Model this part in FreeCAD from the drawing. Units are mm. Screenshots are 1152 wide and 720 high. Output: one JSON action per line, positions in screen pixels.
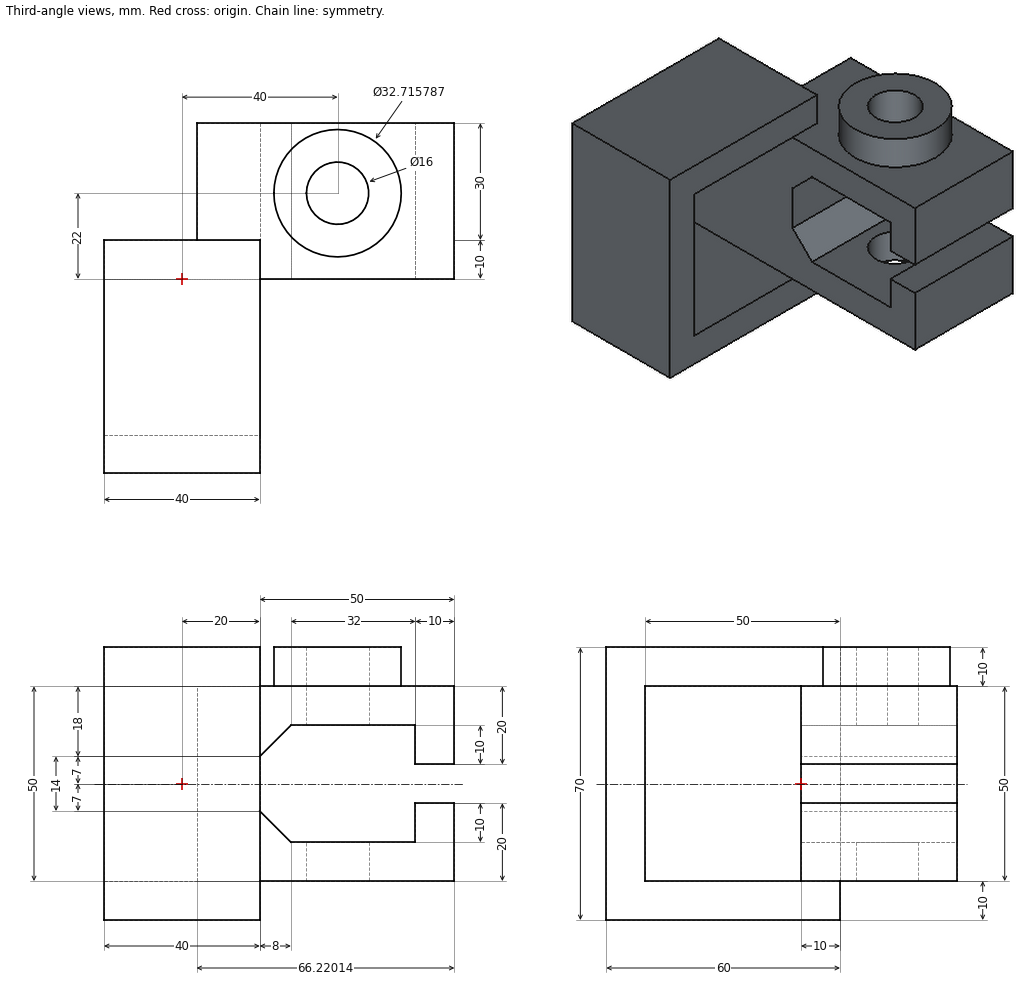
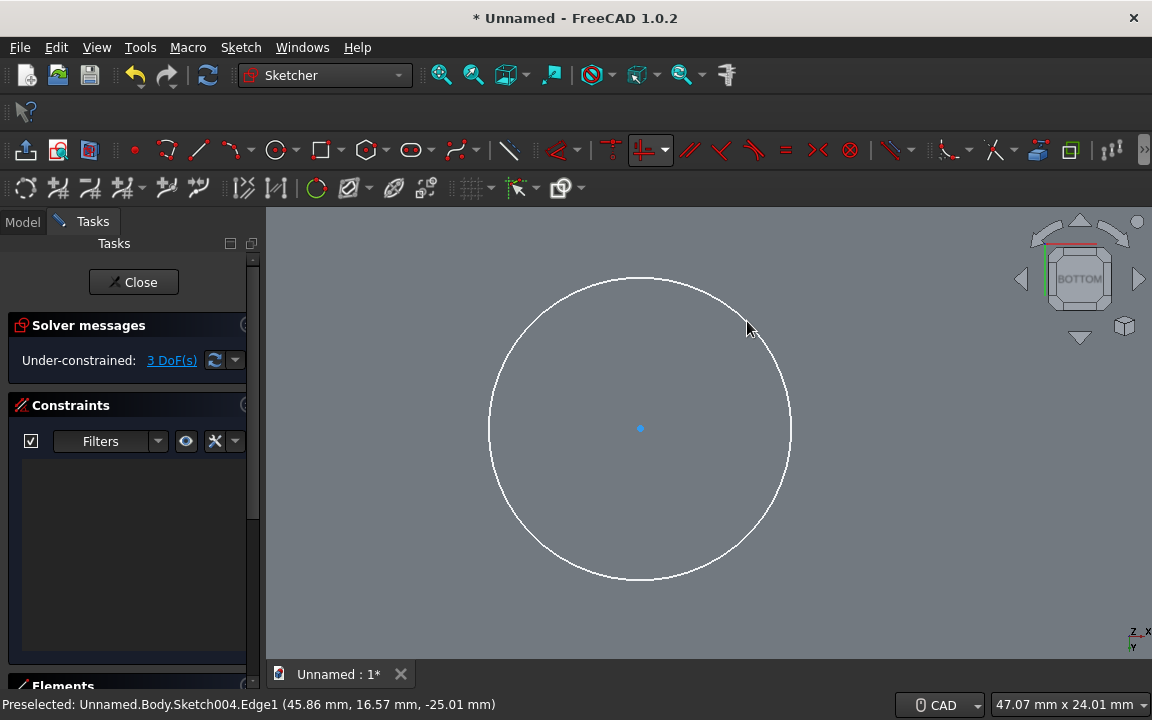
{"action": "key", "text": "d"}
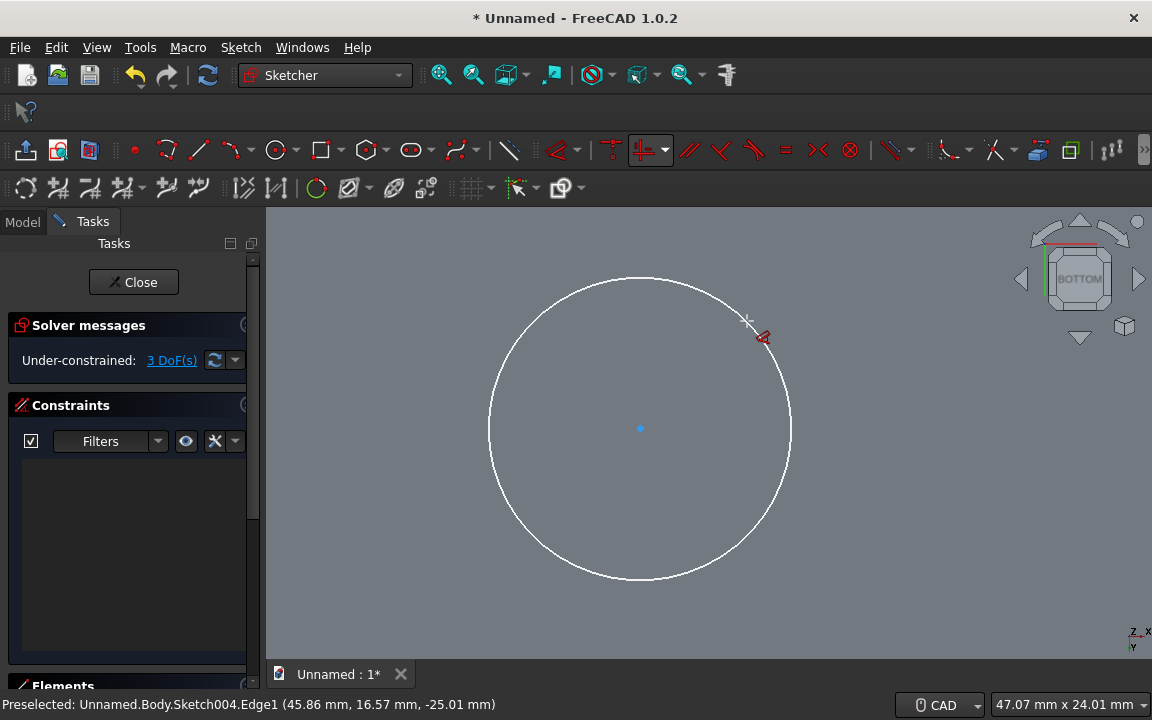
{"action": "left_click", "coordinate": [747, 322]}
{"action": "left_click", "coordinate": [770, 299]}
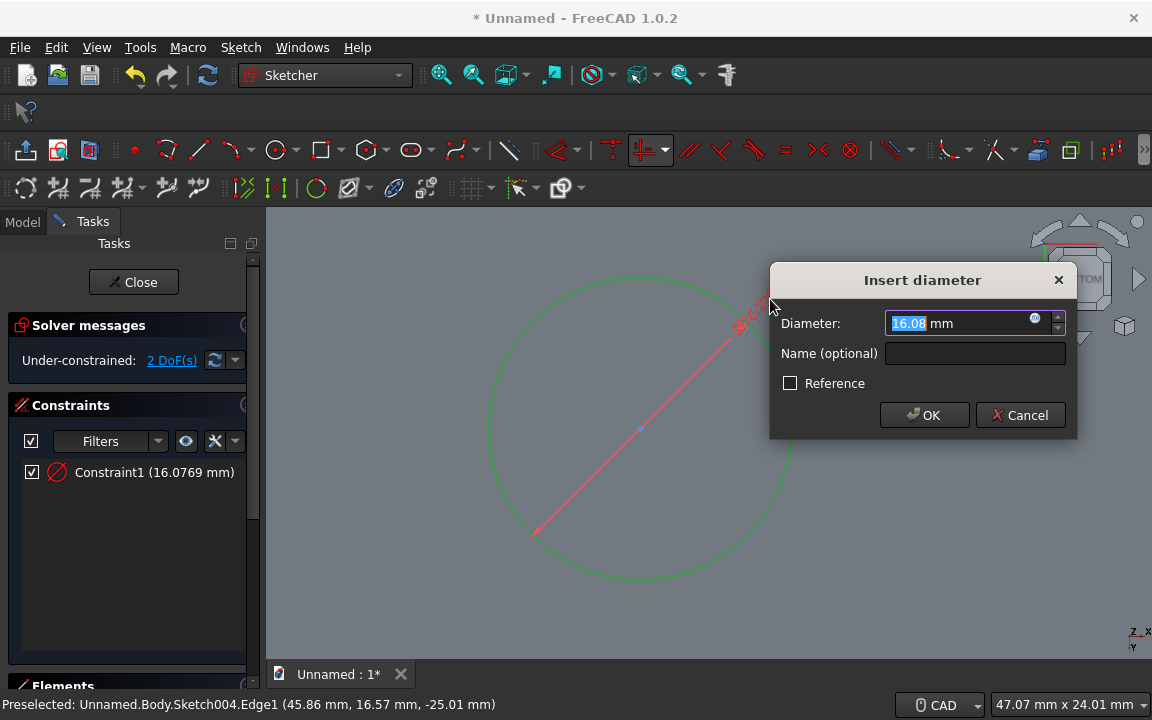
{"action": "type", "text": "16"}
{"action": "key", "text": "Return"}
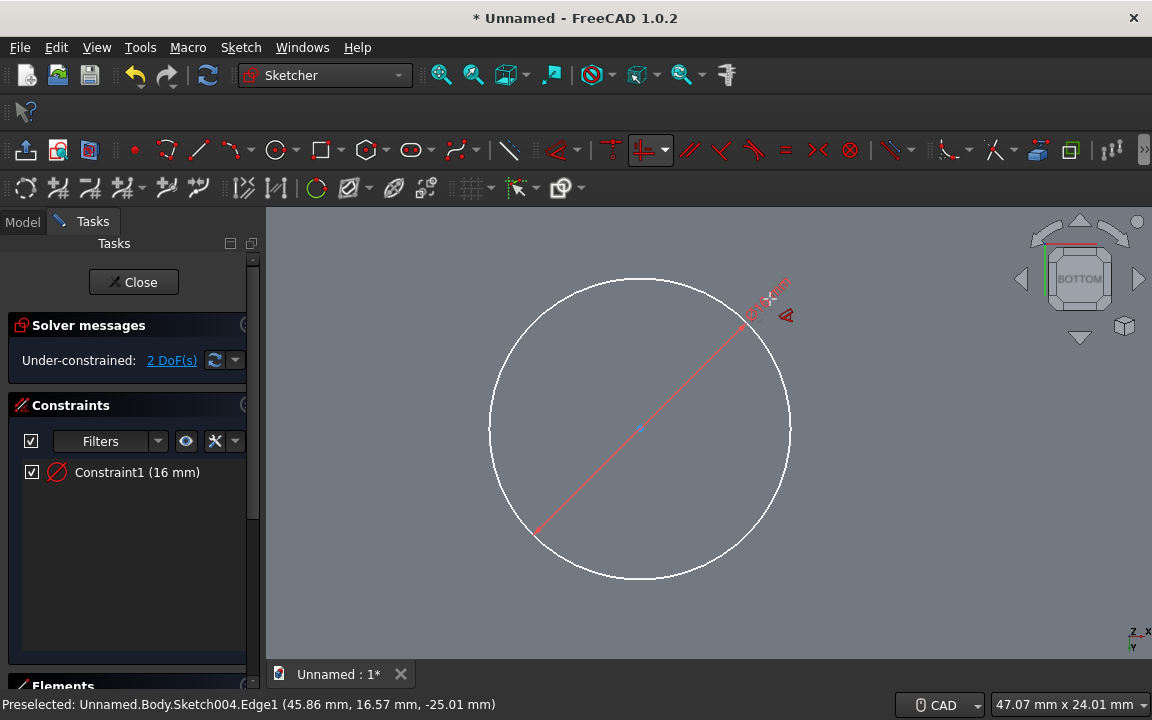
{"action": "left_click", "coordinate": [640, 429]}
{"action": "left_click", "coordinate": [467, 463]}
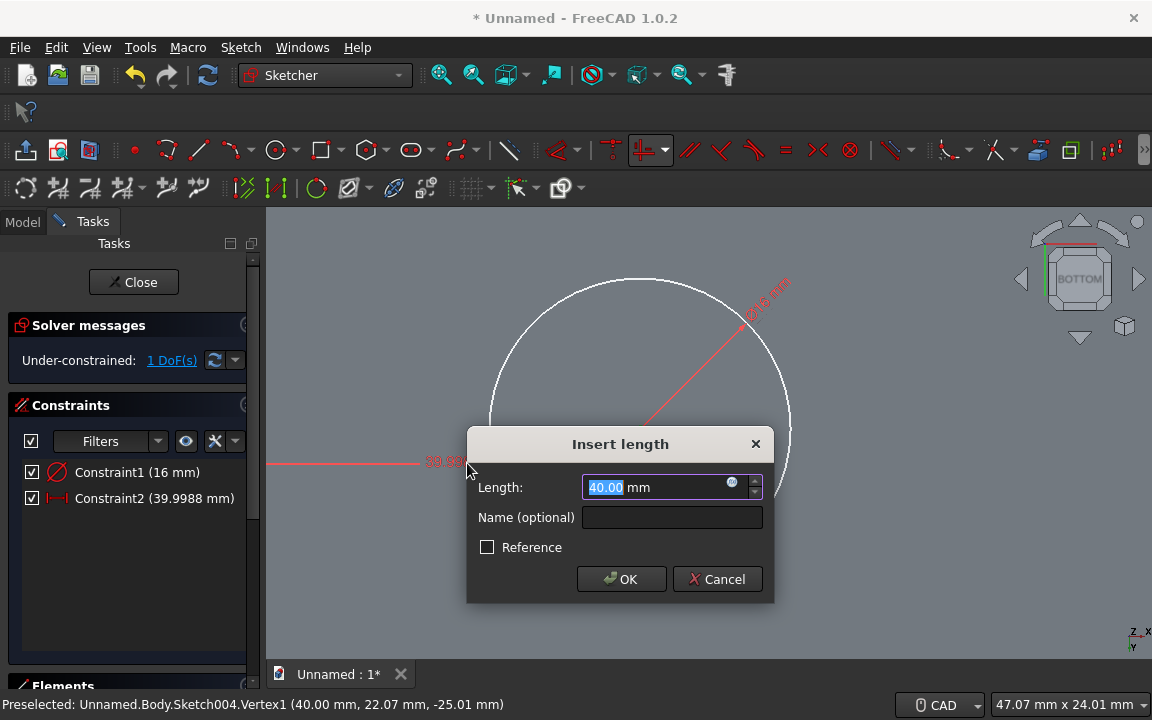
{"action": "type", "text": "40"}
{"action": "key", "text": "Return"}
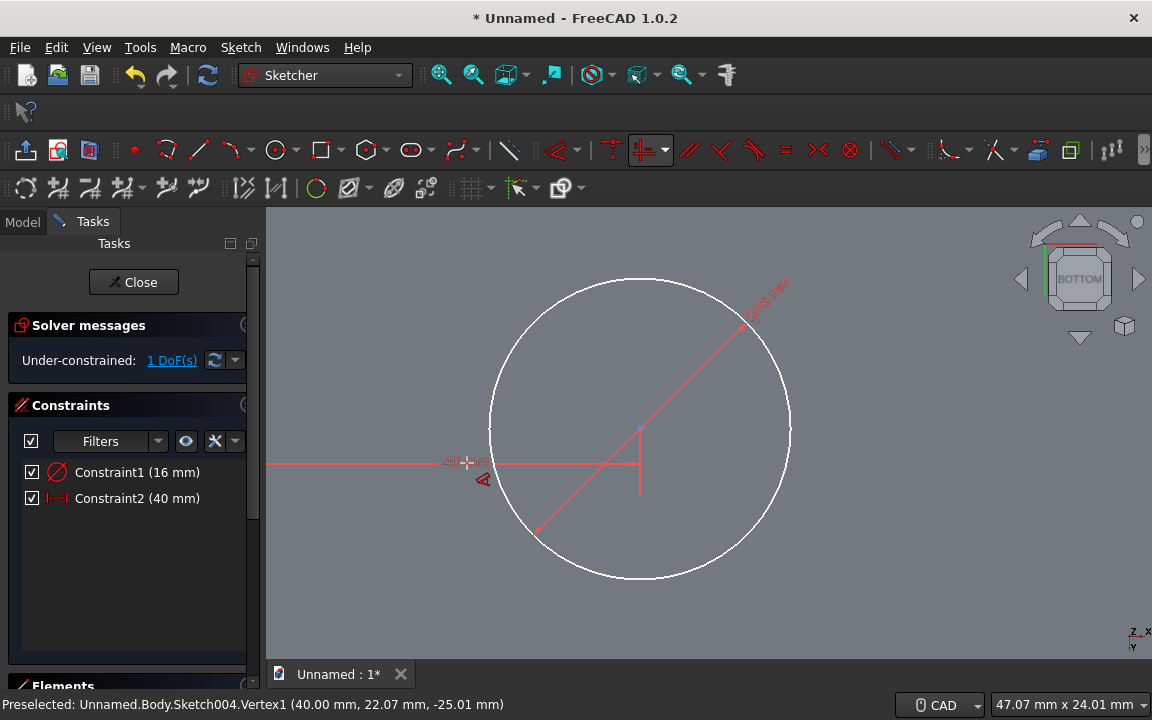
{"action": "left_click", "coordinate": [640, 429]}
{"action": "left_click", "coordinate": [674, 332]}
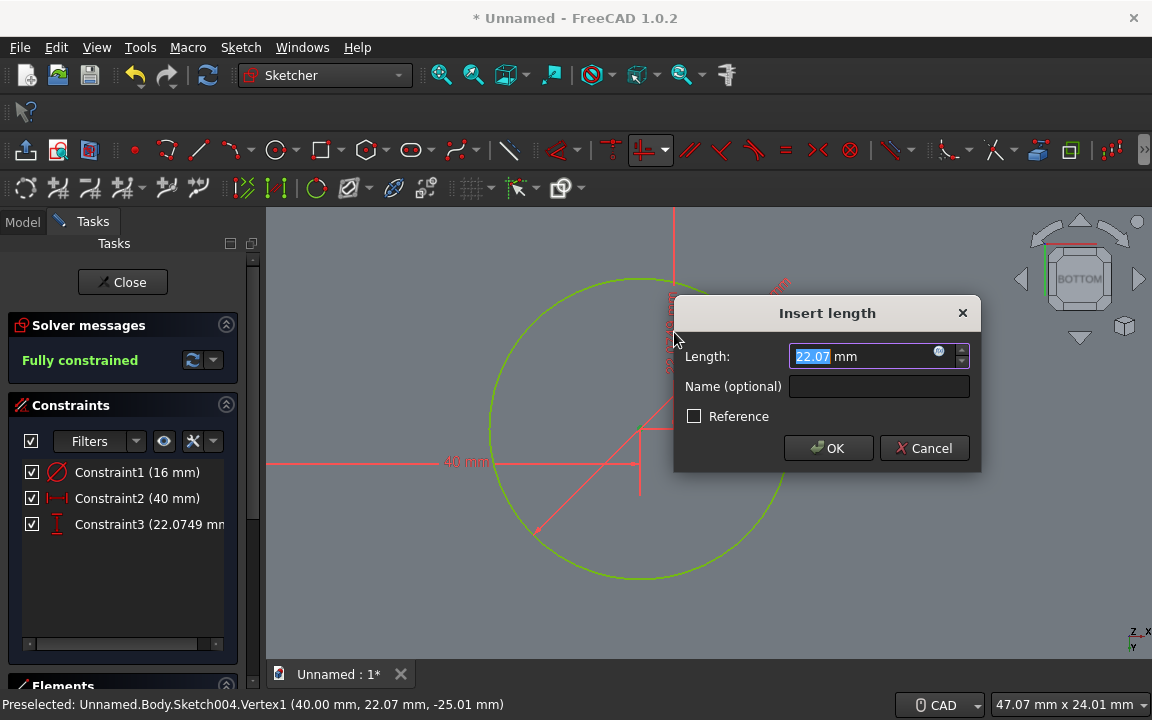
{"action": "type", "text": "22"}
{"action": "key", "text": "Return"}
{"action": "key", "text": "Escape"}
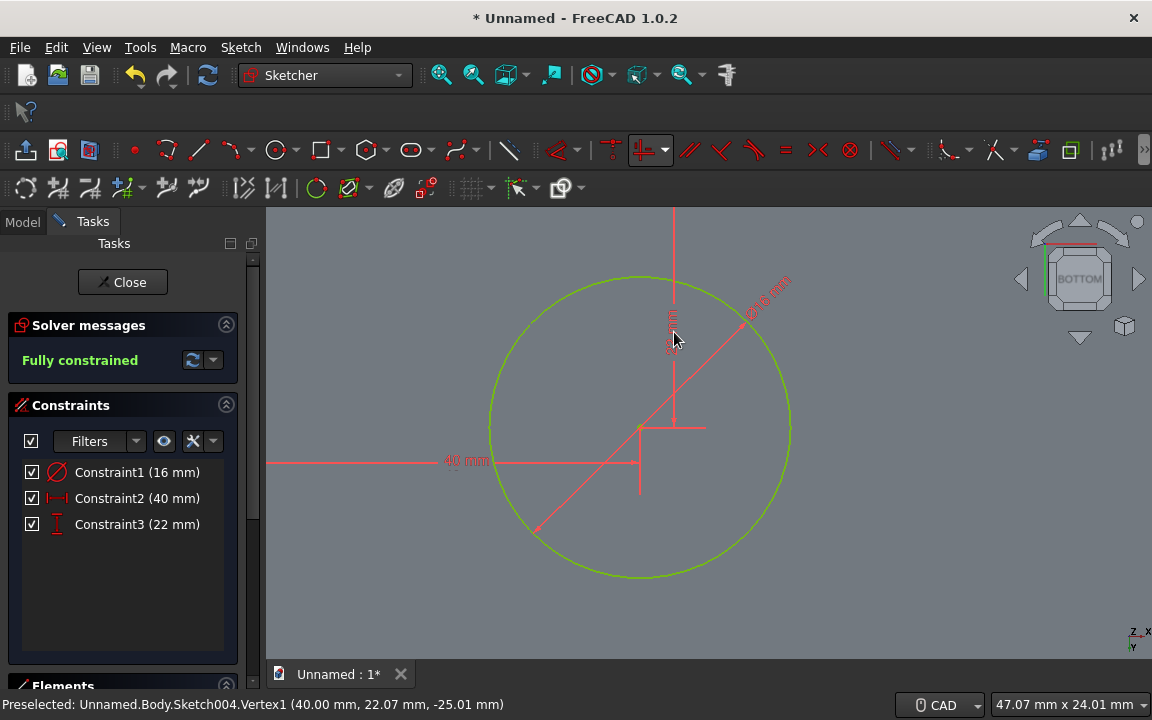
{"action": "left_click", "coordinate": [123, 282]}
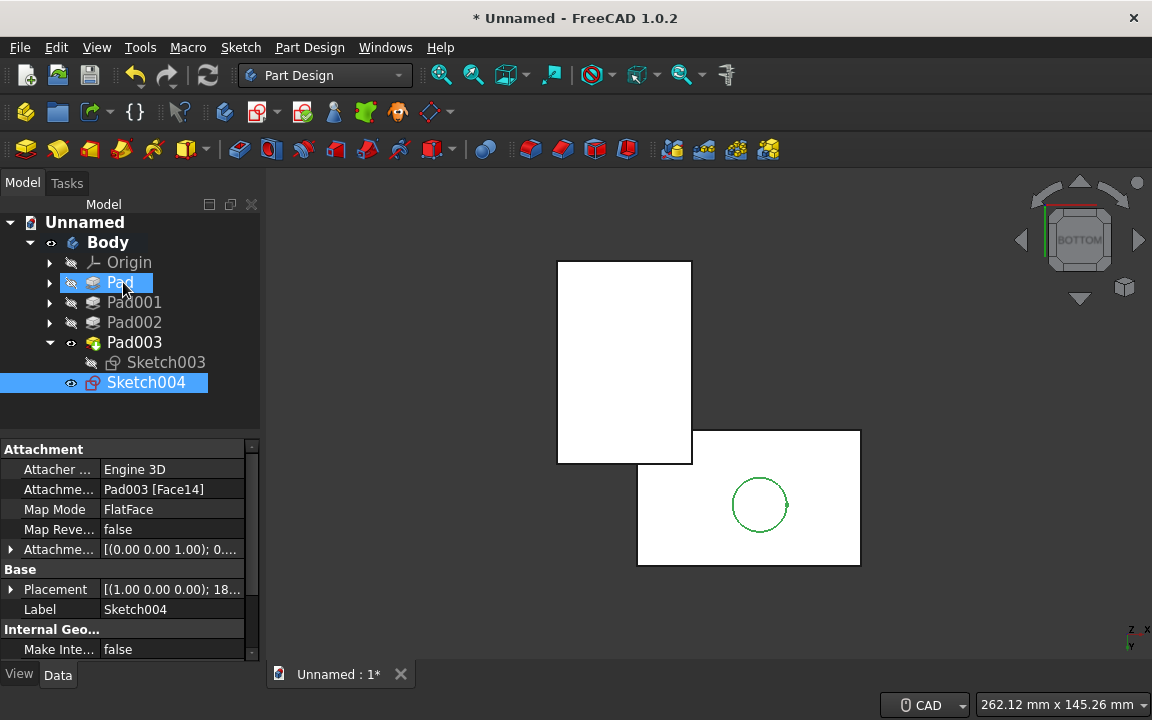
{"action": "left_click", "coordinate": [240, 150]}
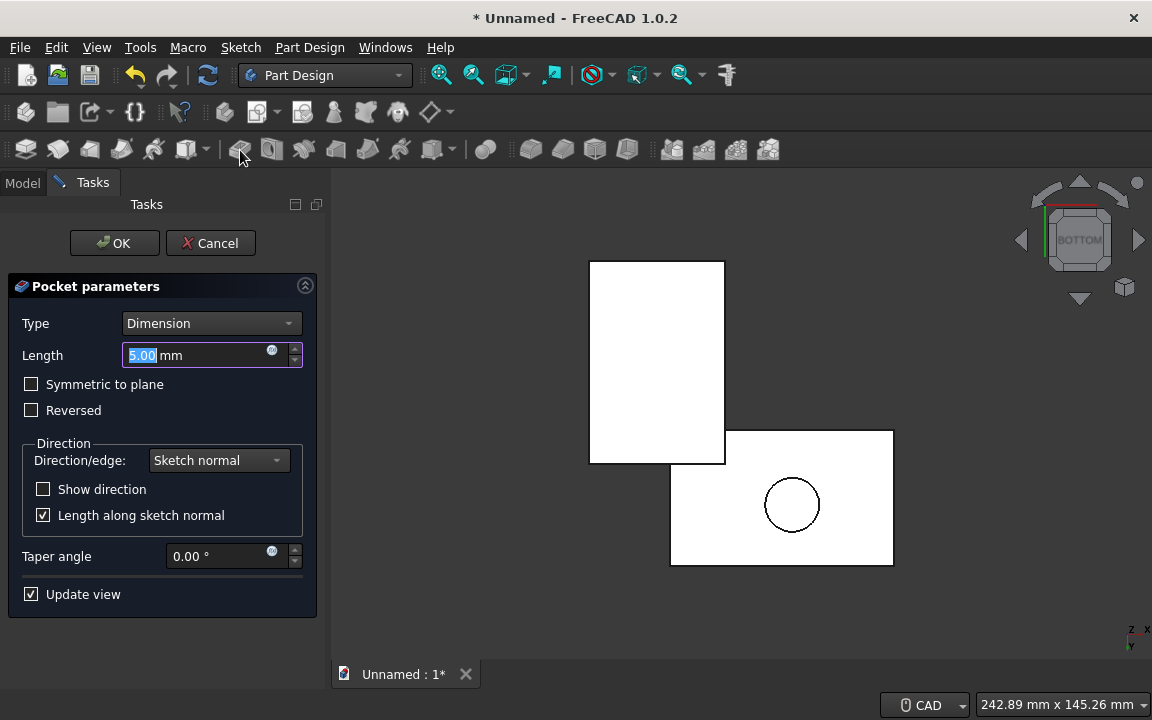
{"action": "type", "text": "50"}
{"action": "key", "text": "Tab"}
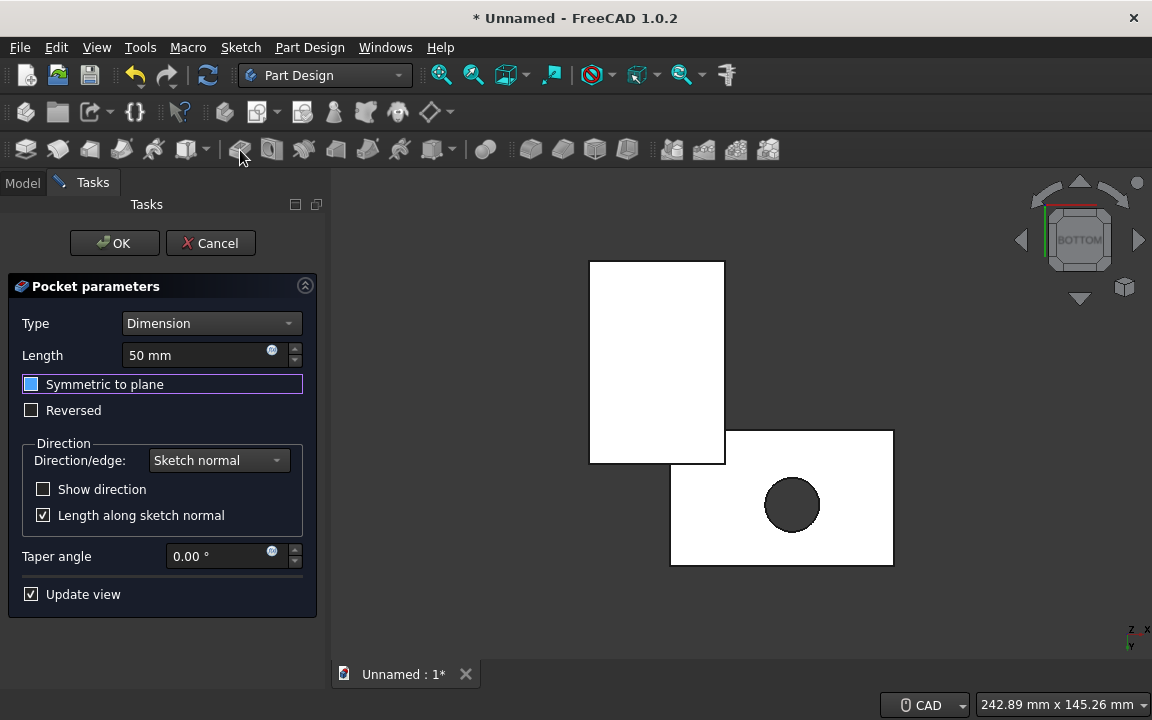
{"action": "left_click", "coordinate": [115, 243]}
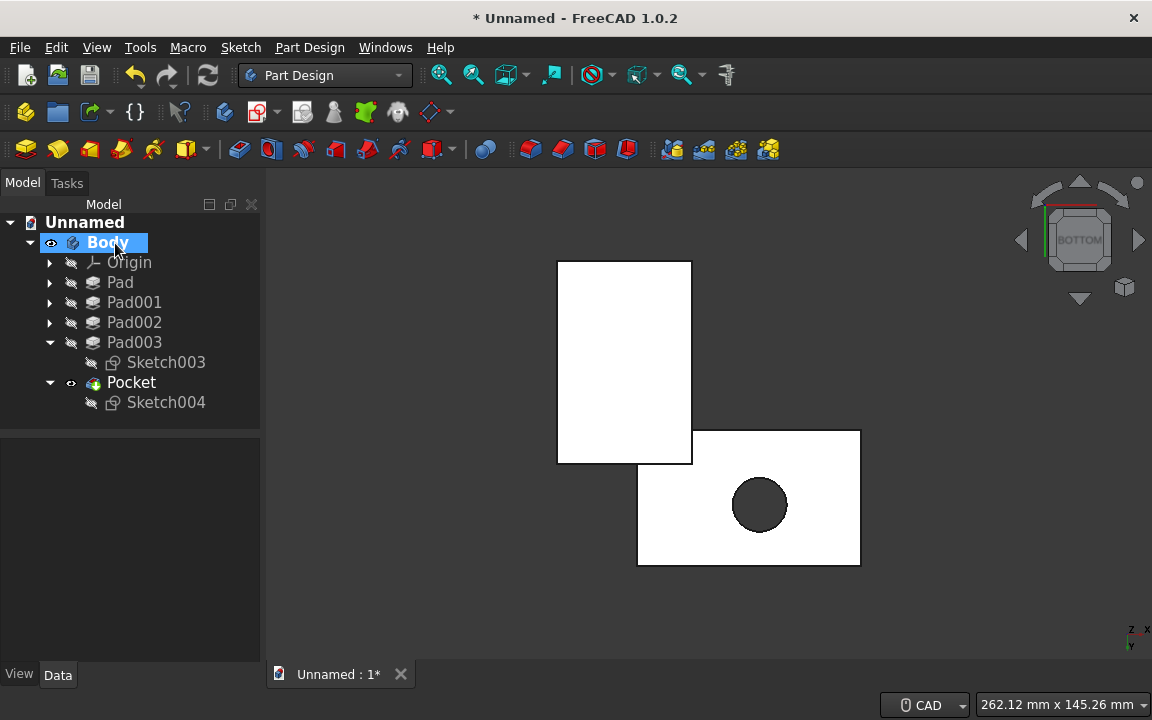
{"action": "key", "text": "0"}